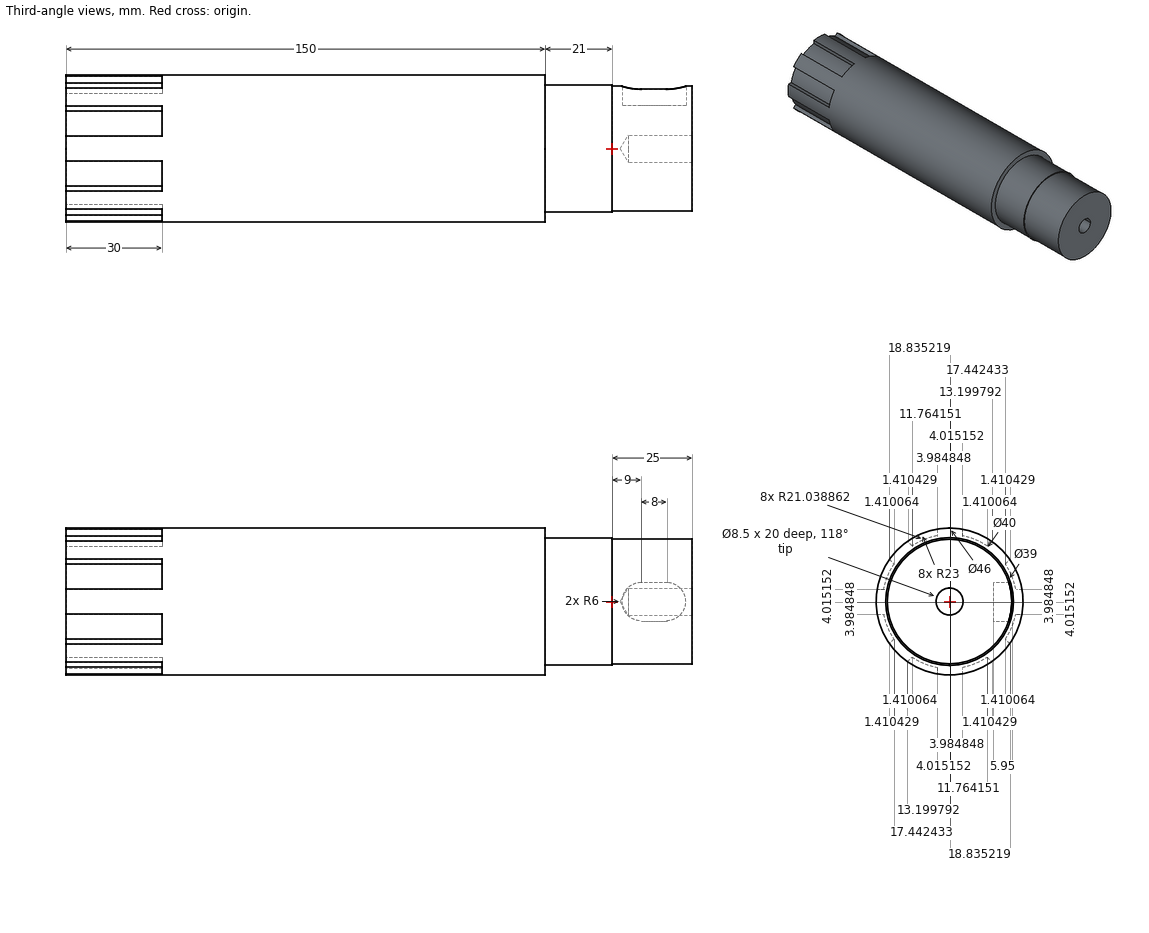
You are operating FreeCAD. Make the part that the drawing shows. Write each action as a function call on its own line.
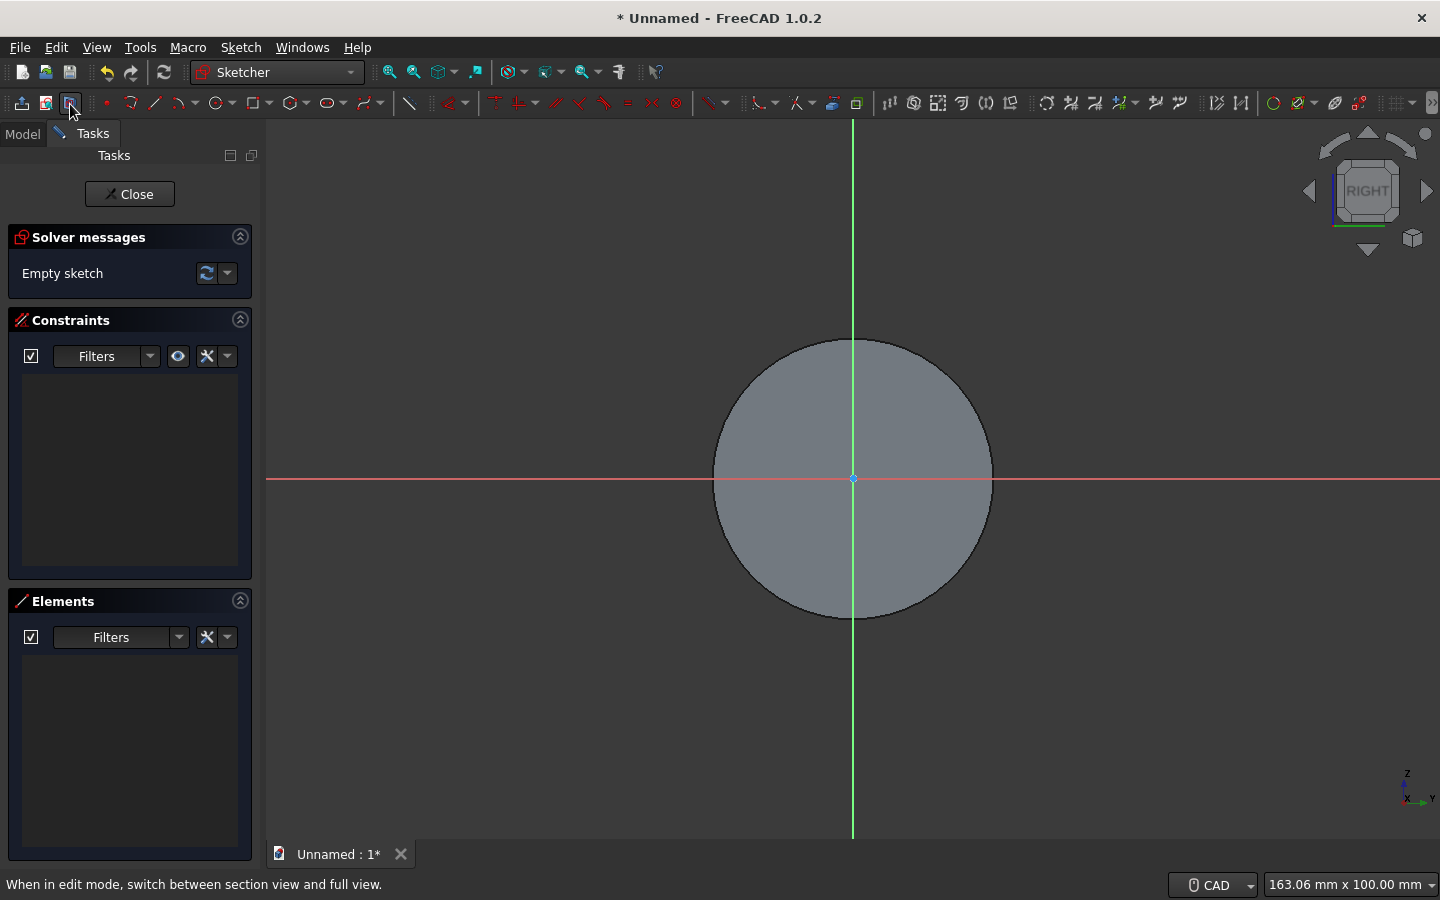
scroll(992, 479, up, 2)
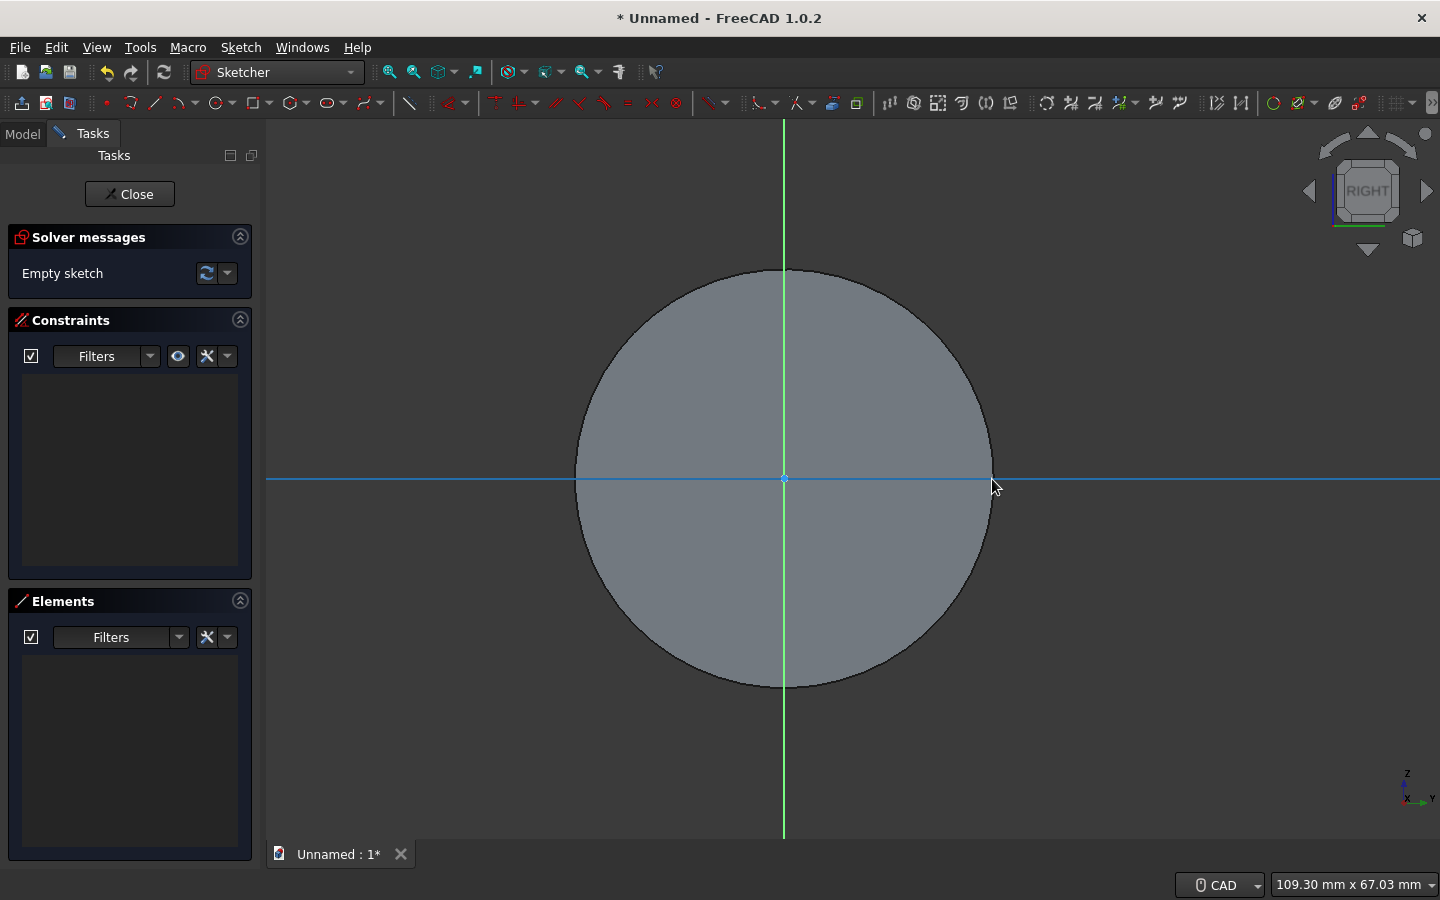
click(216, 104)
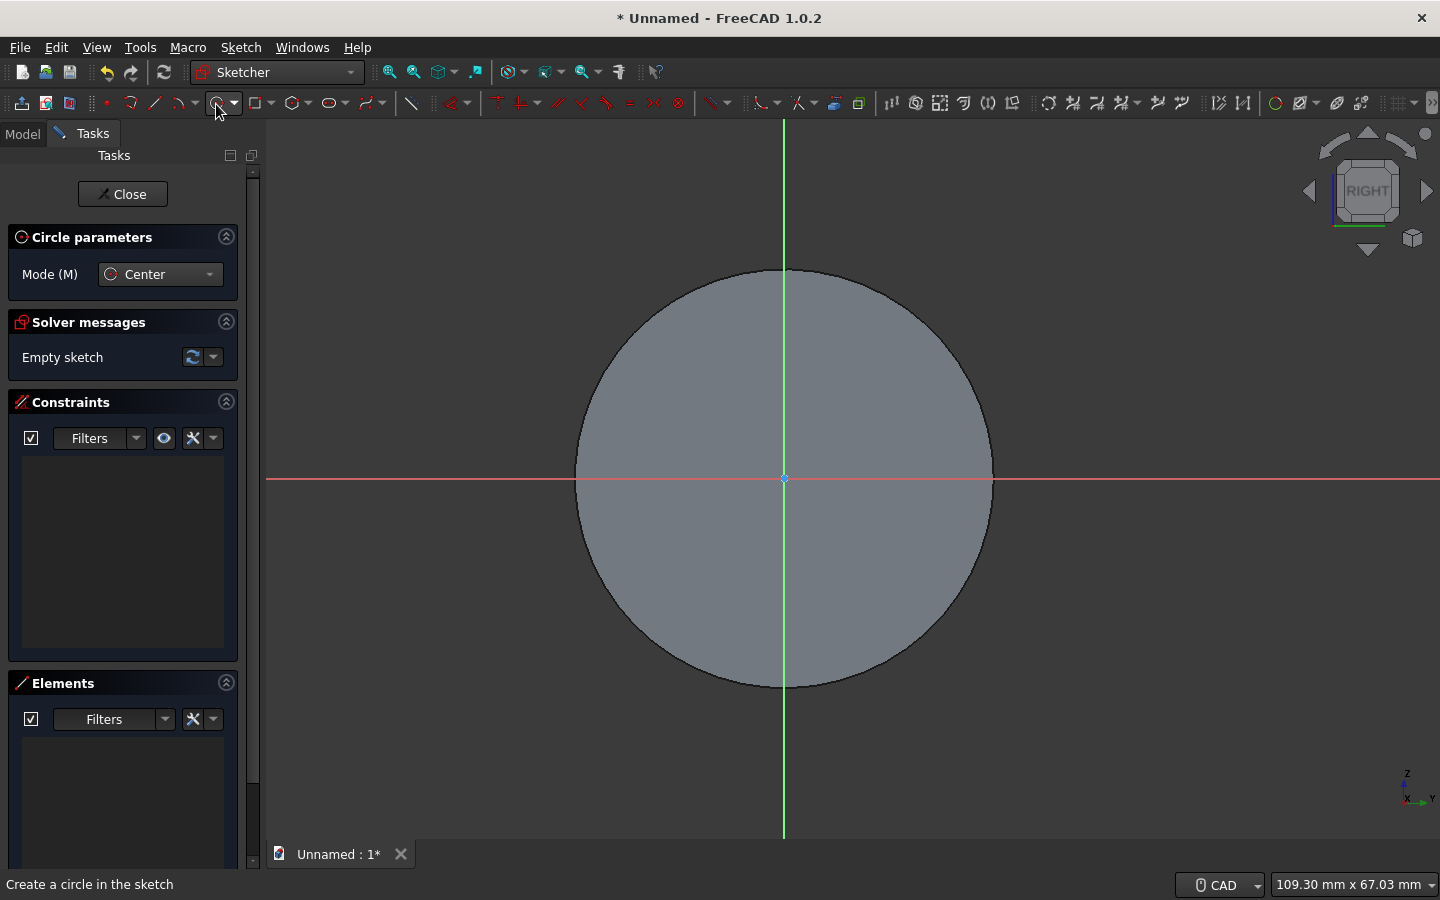
click(784, 479)
click(936, 327)
key(Escape)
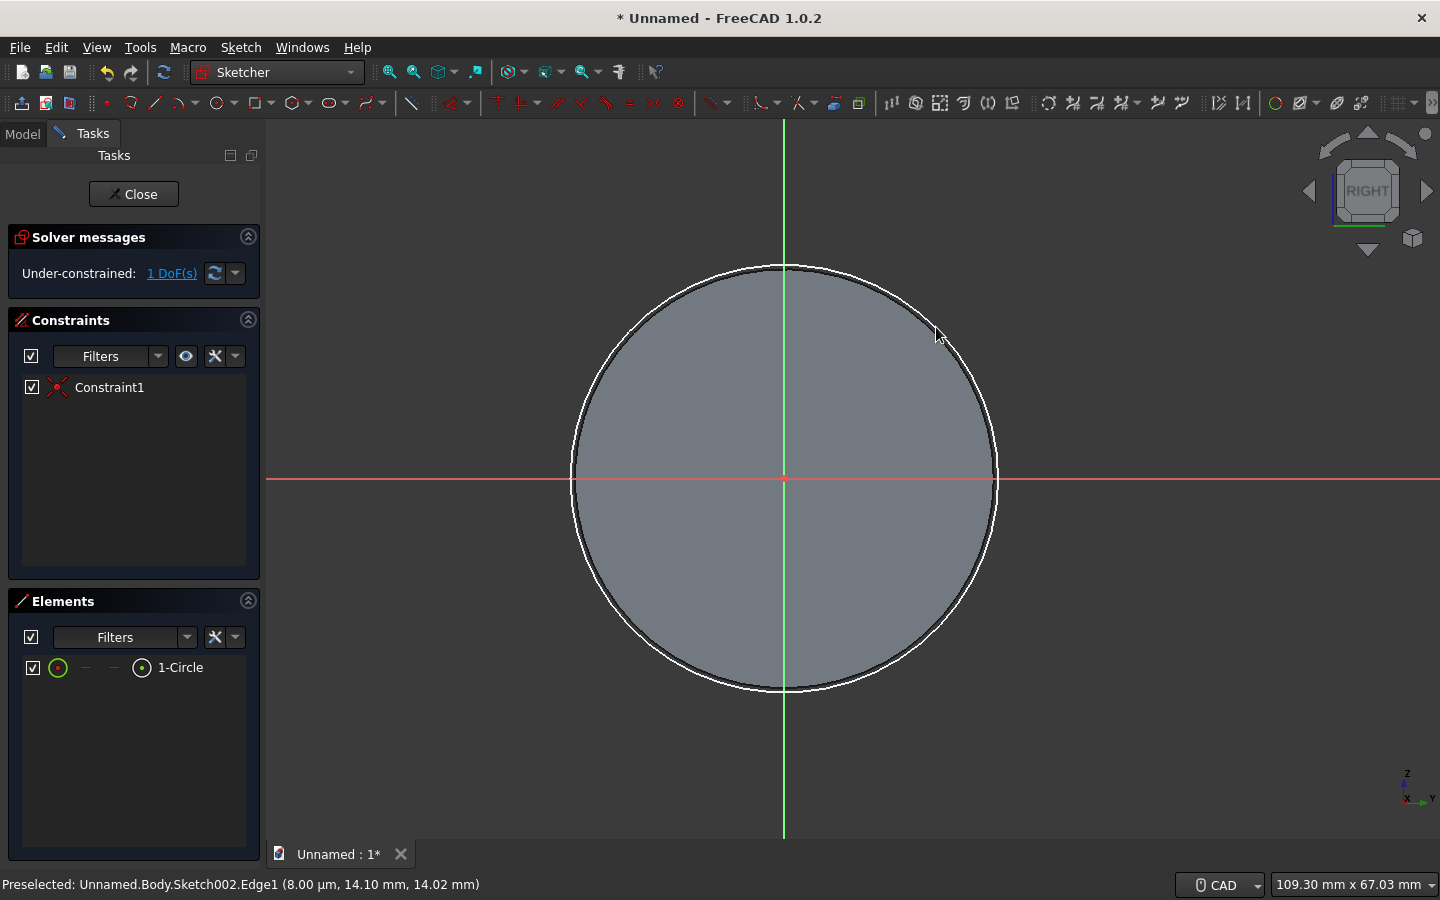
click(450, 104)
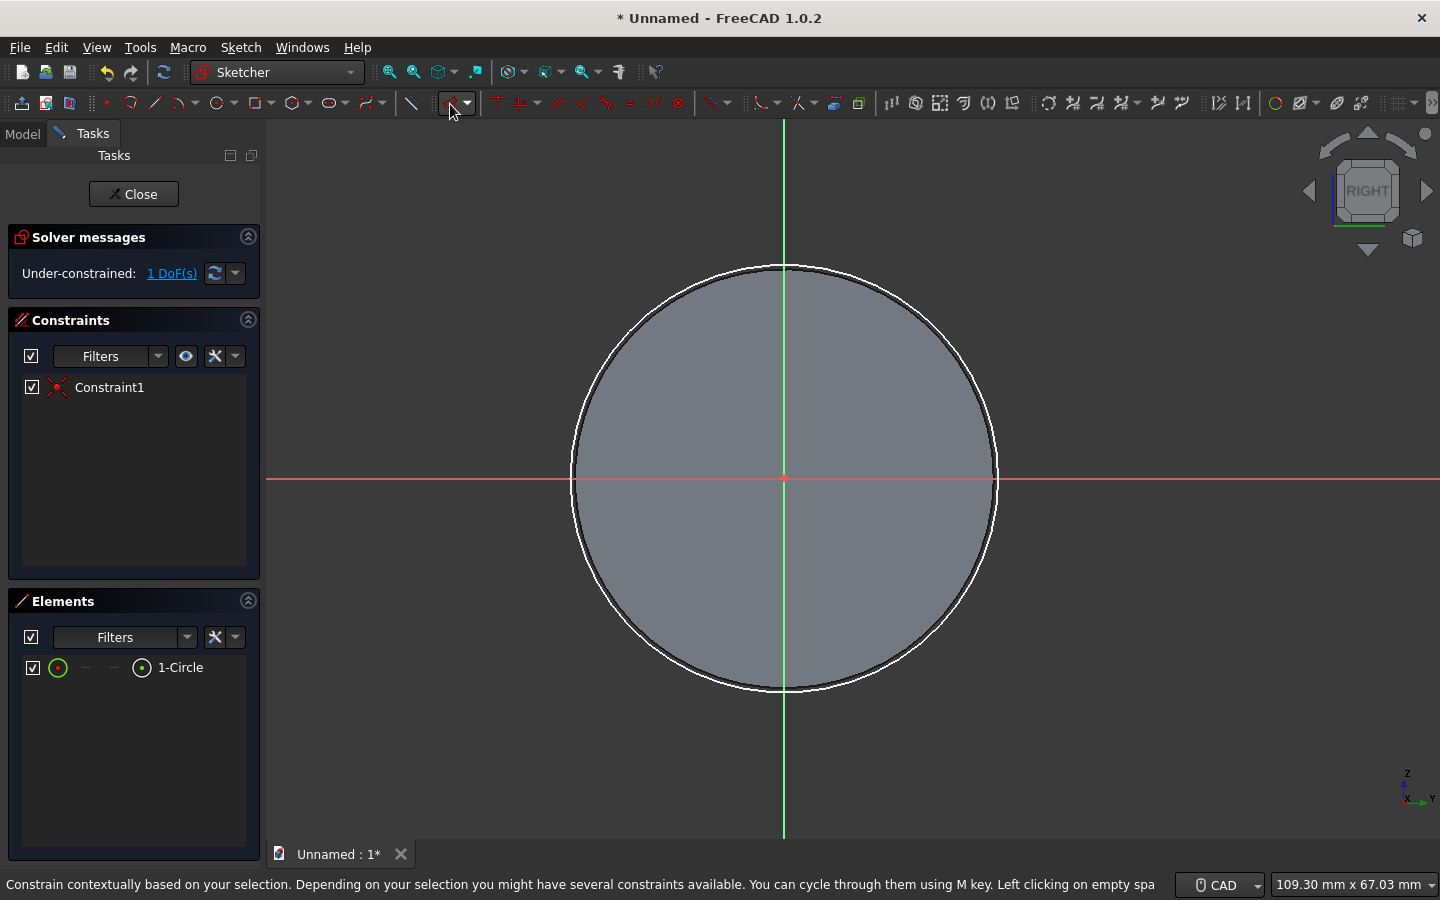
click(935, 327)
click(958, 304)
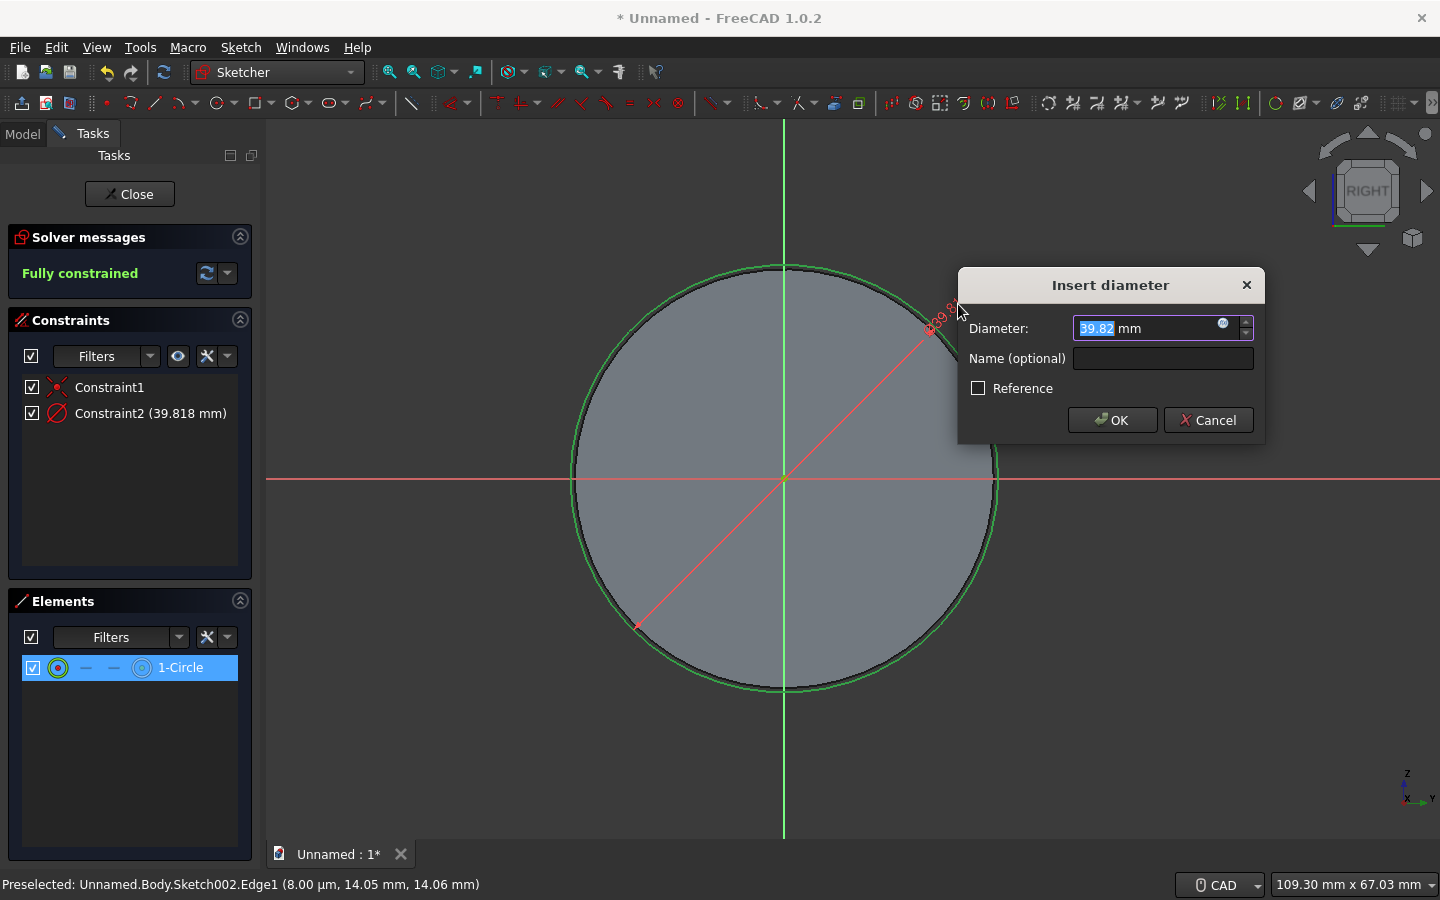
text(40)
key(Return)
key(Escape)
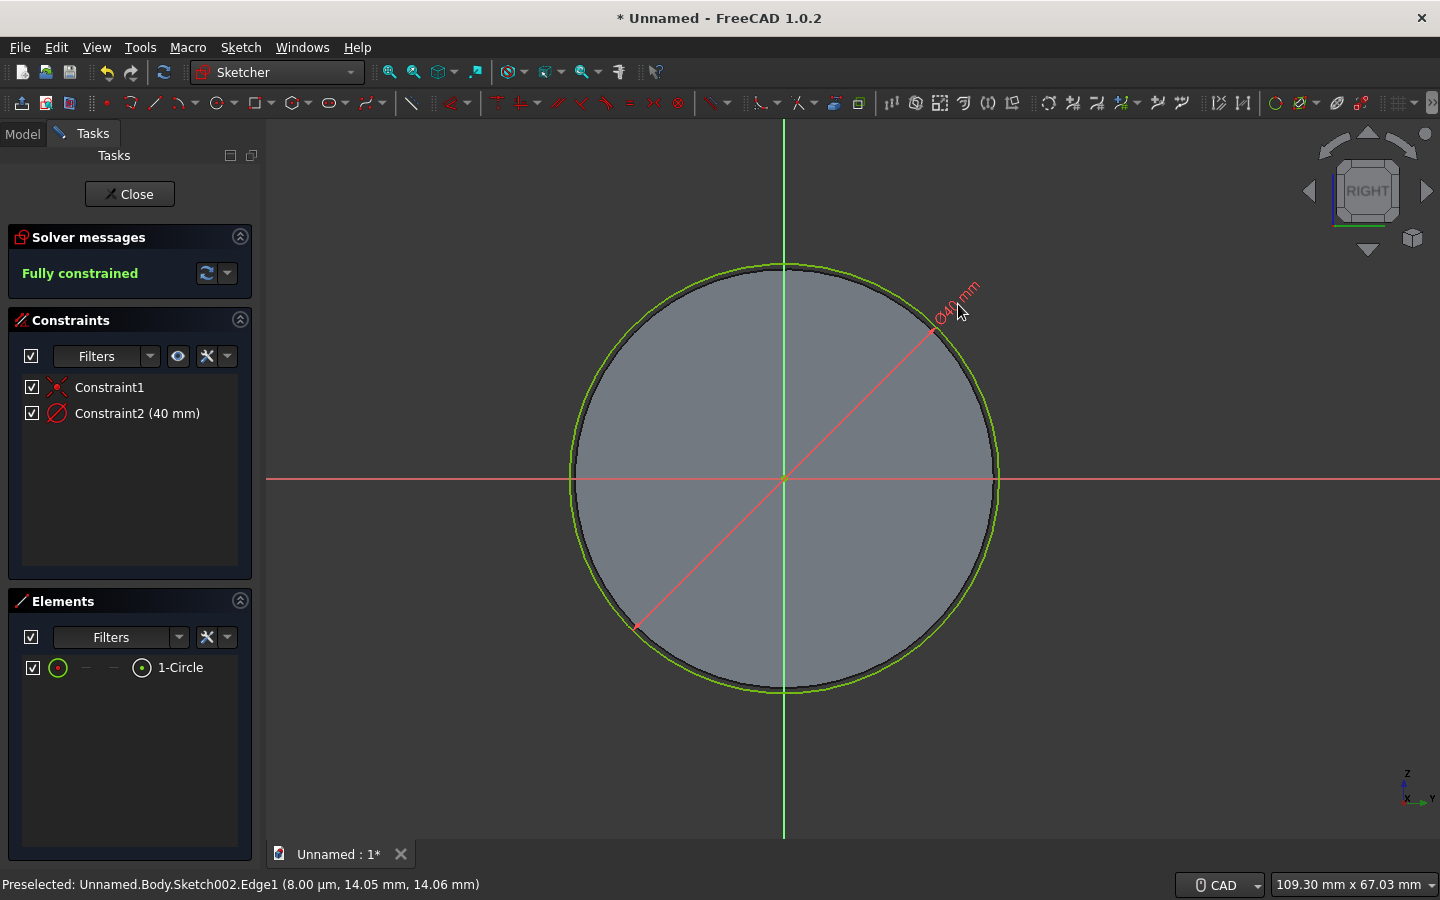
click(130, 194)